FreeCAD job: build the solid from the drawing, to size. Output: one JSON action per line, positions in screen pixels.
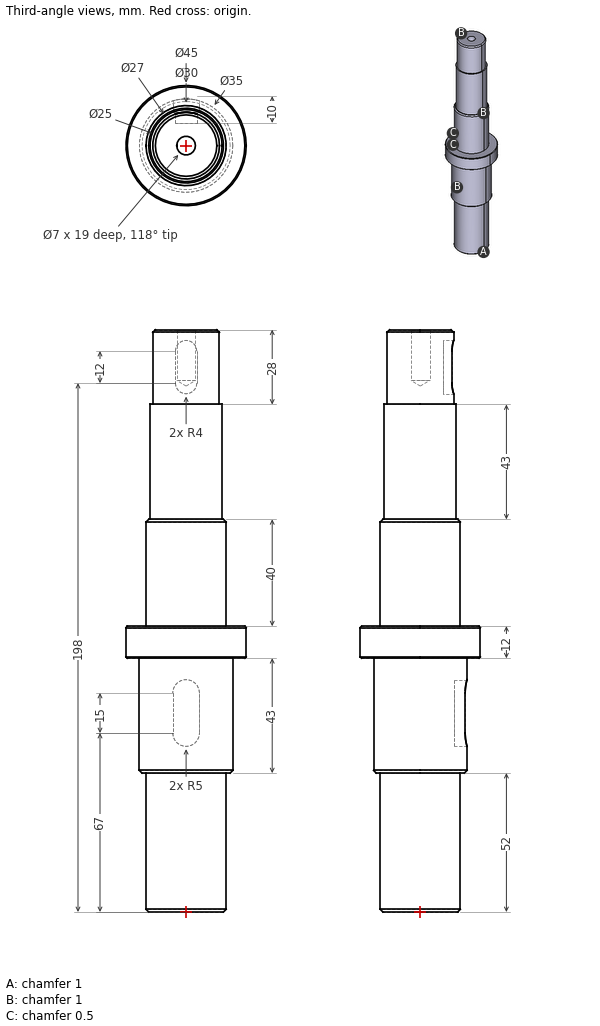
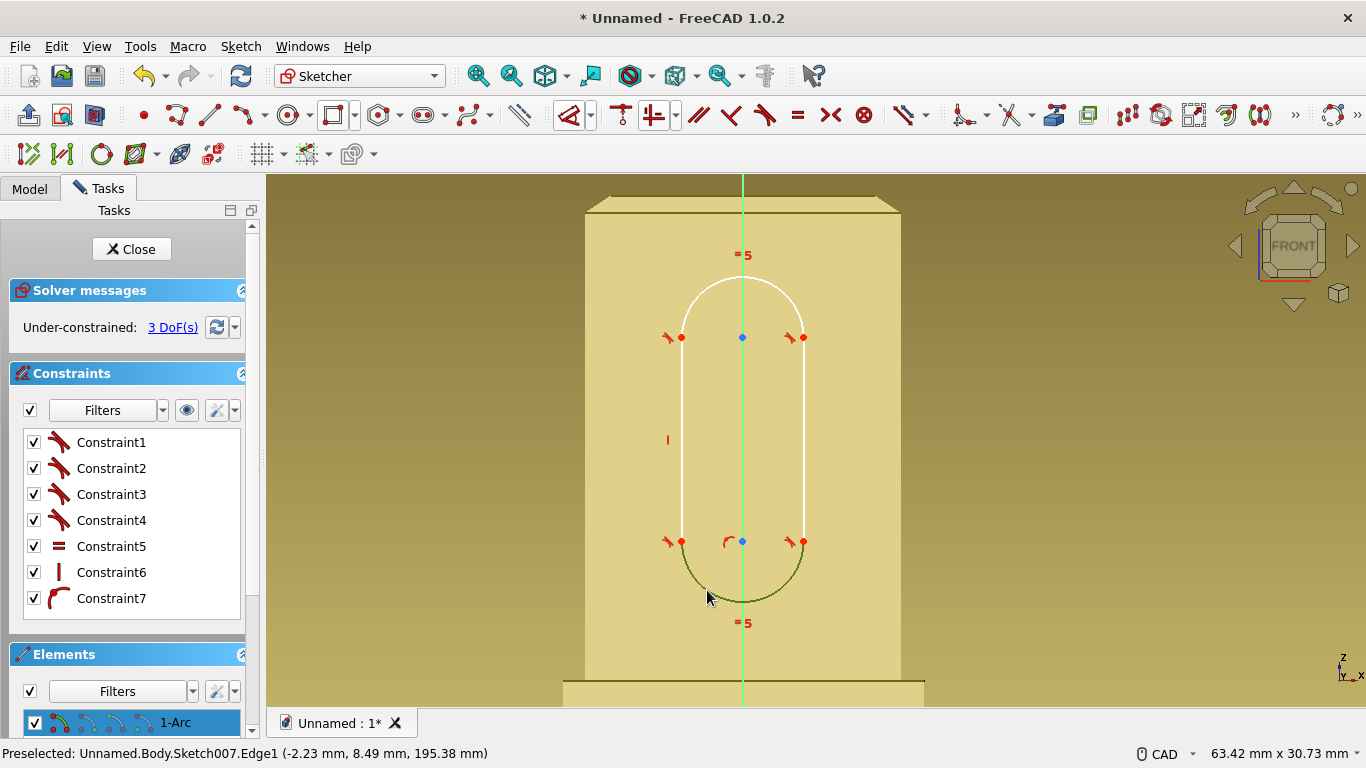
{"action": "key", "text": "k r"}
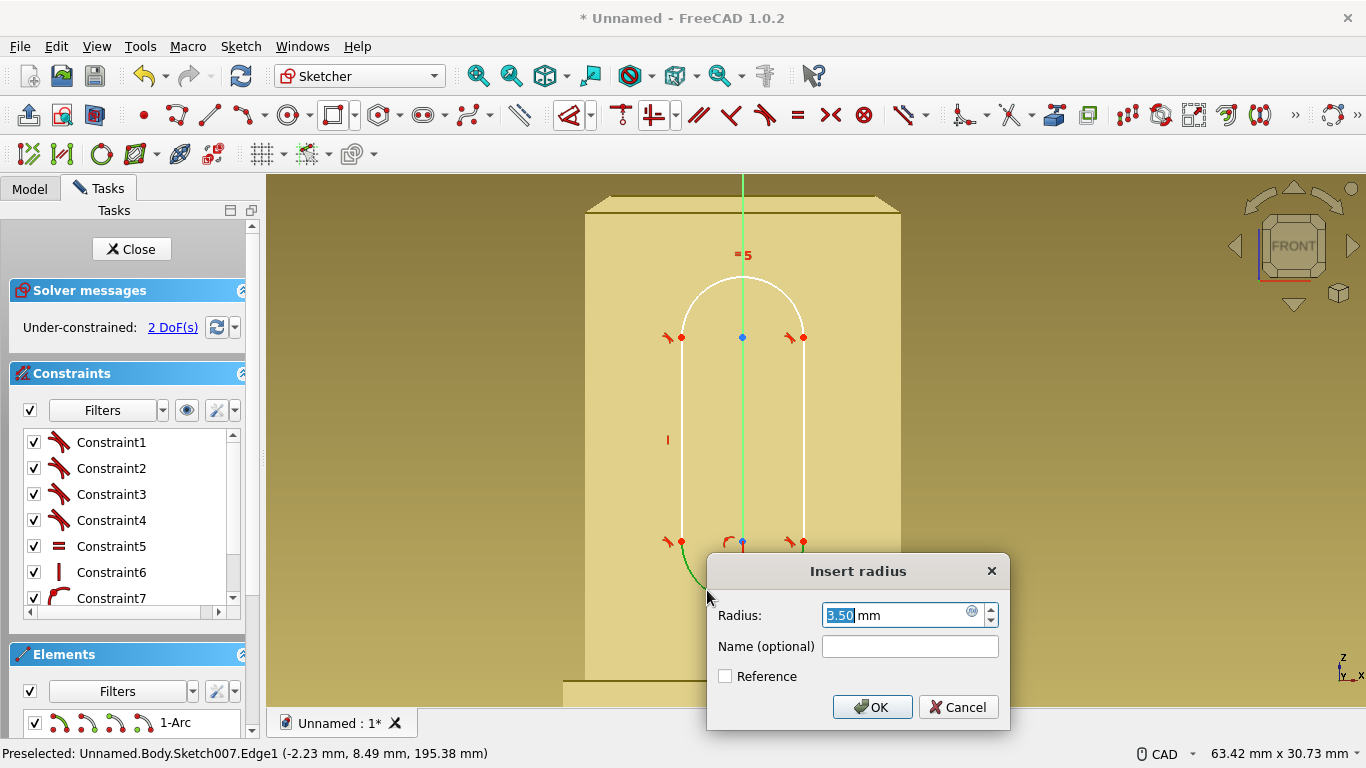
{"action": "type", "text": "4"}
{"action": "key", "text": "Return"}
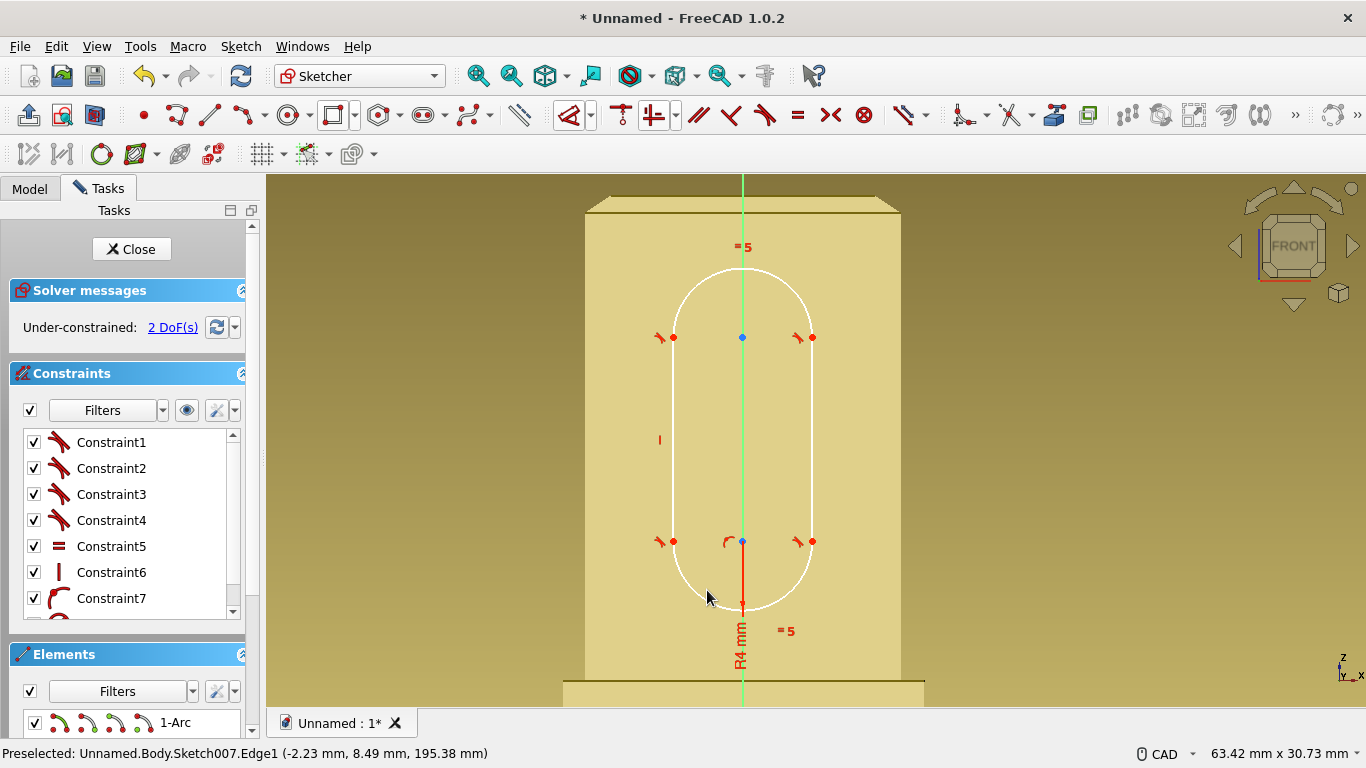
{"action": "left_click", "coordinate": [673, 480]}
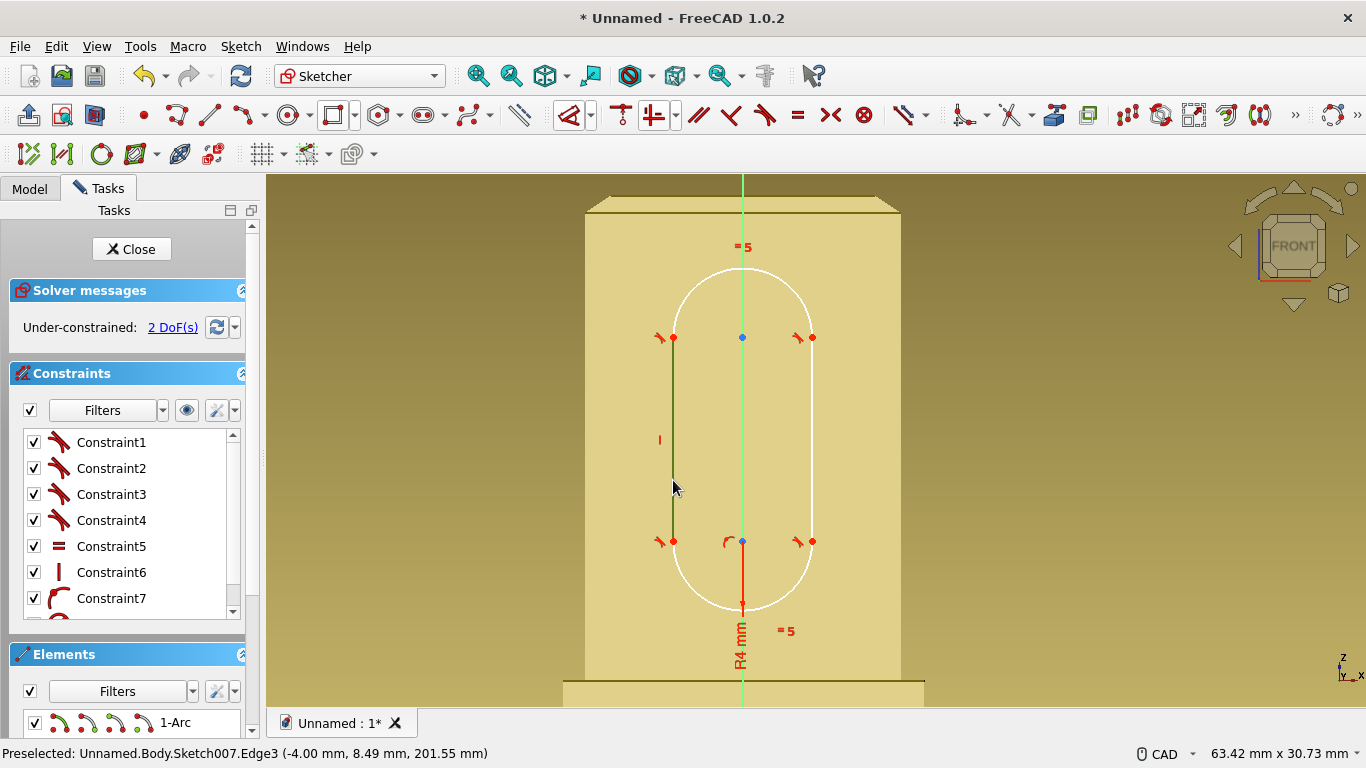
{"action": "key", "text": "i"}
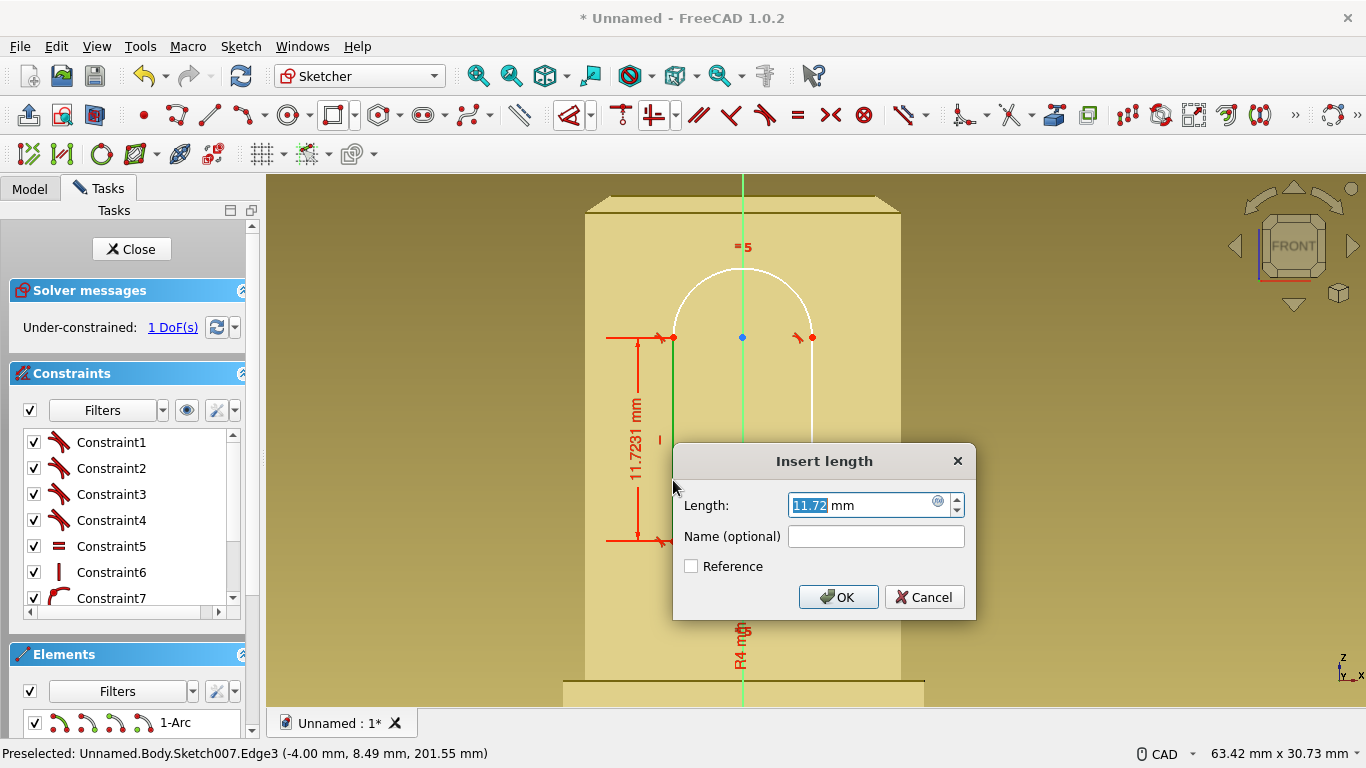
{"action": "type", "text": "12"}
{"action": "key", "text": "Return"}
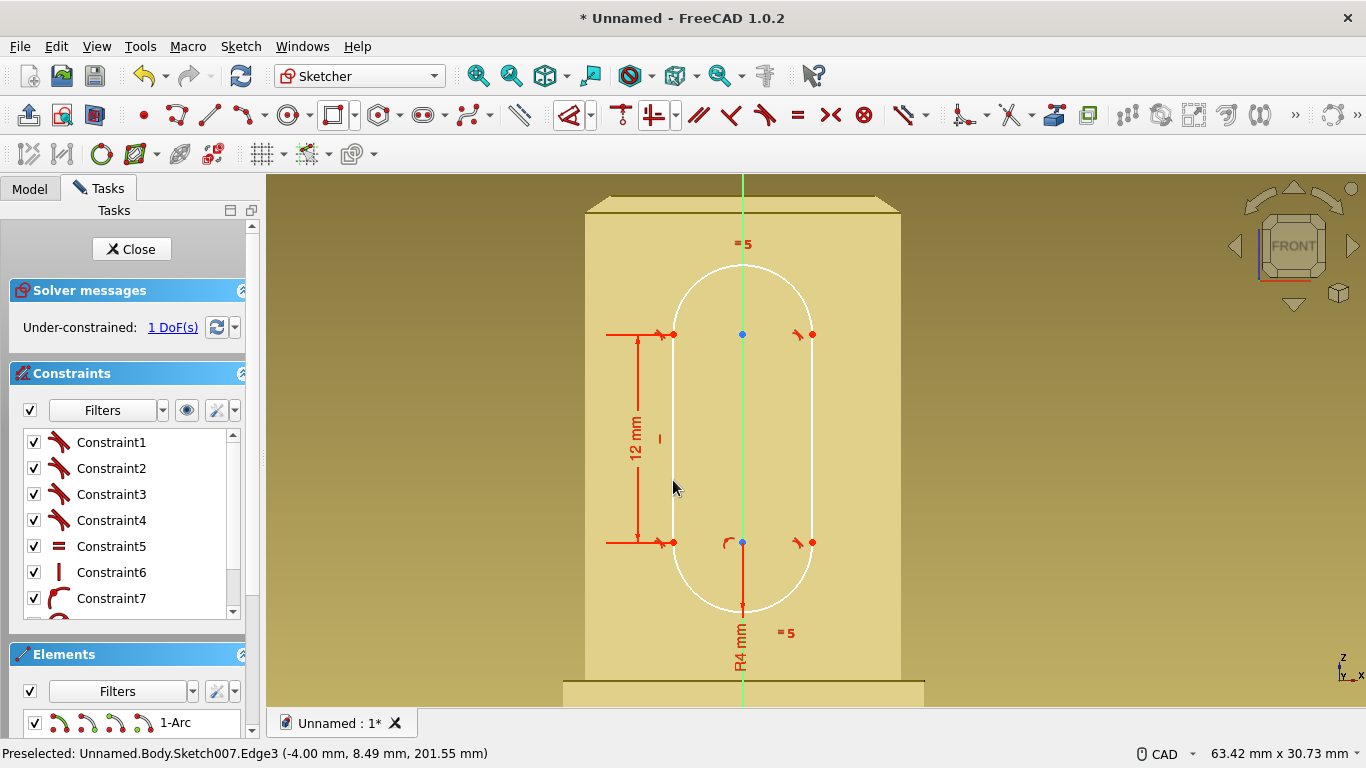
{"action": "left_click", "coordinate": [673, 543]}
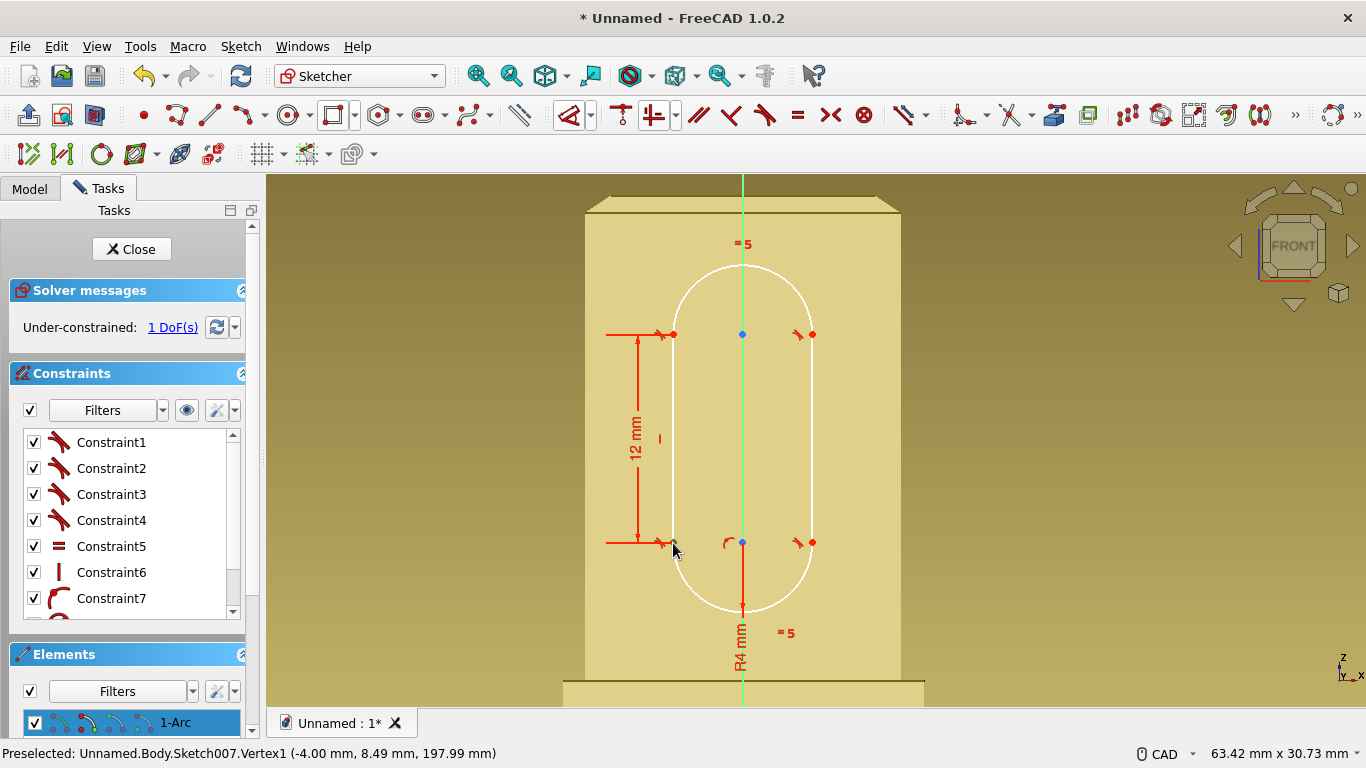
{"action": "key", "text": "i"}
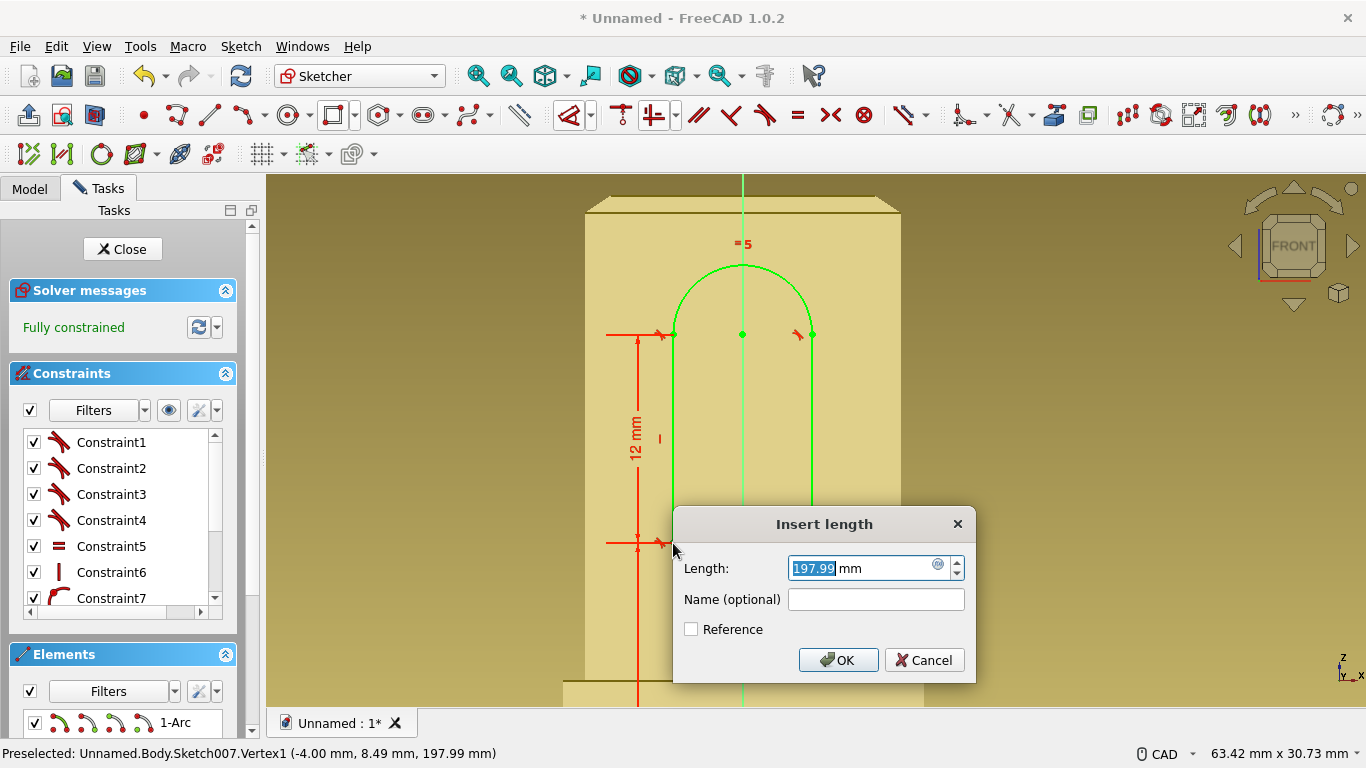
{"action": "type", "text": "198"}
{"action": "key", "text": "Return"}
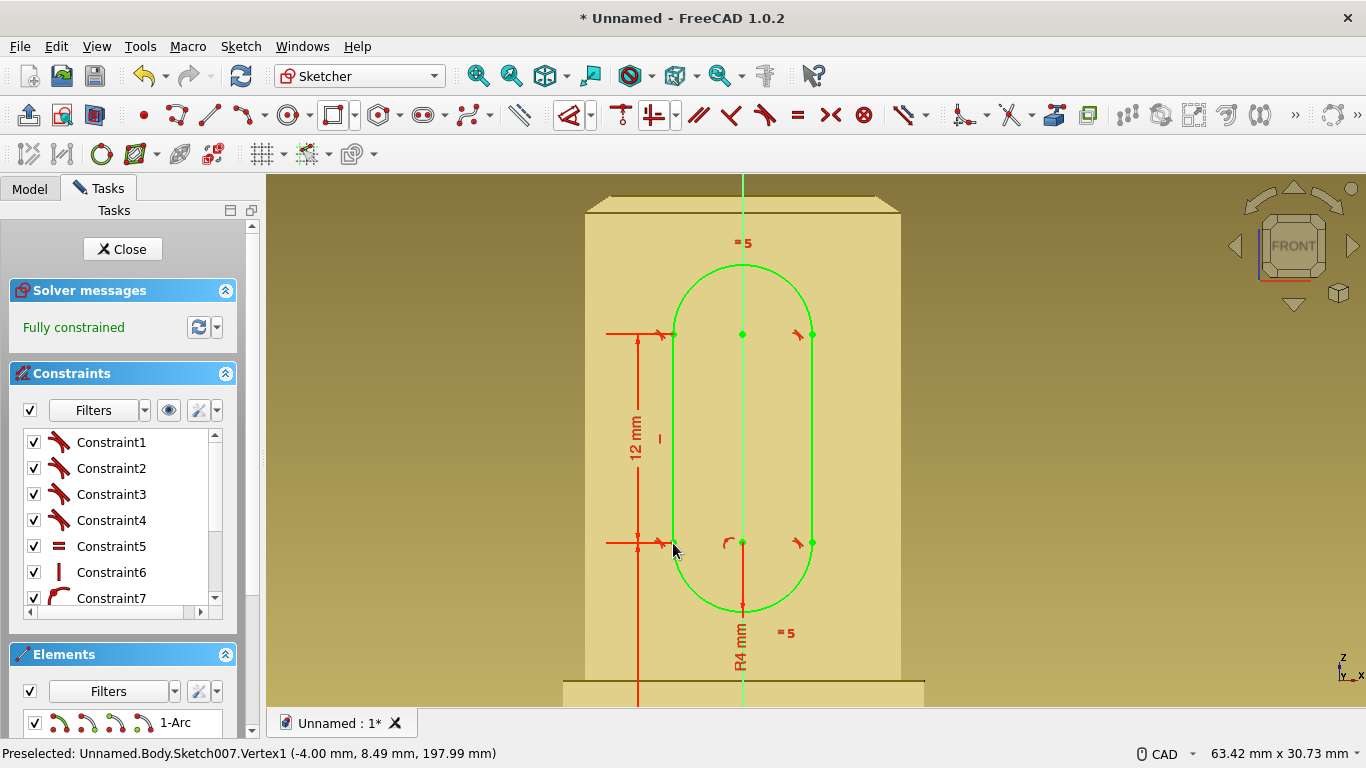
{"action": "left_click", "coordinate": [123, 249]}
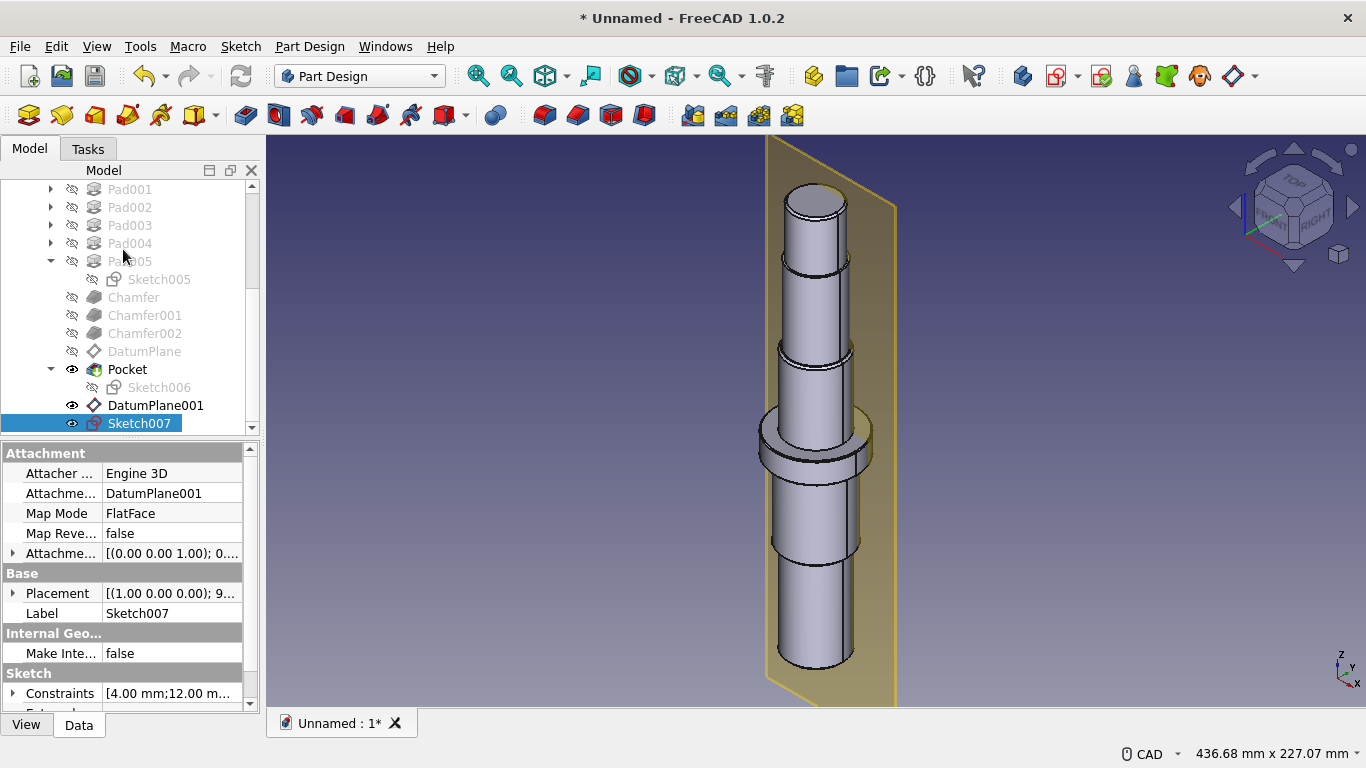
{"action": "left_click", "coordinate": [246, 116]}